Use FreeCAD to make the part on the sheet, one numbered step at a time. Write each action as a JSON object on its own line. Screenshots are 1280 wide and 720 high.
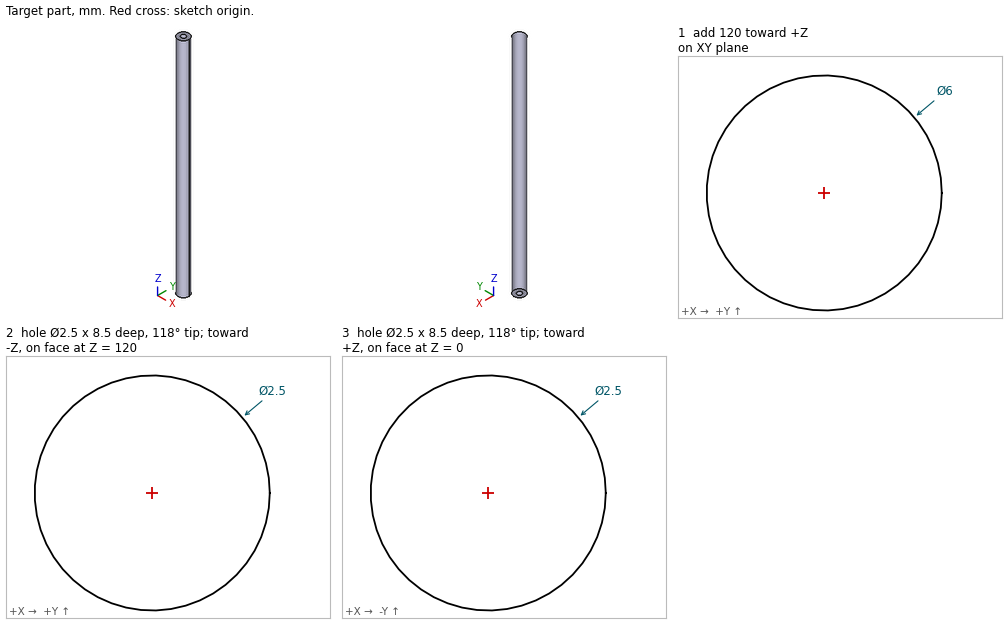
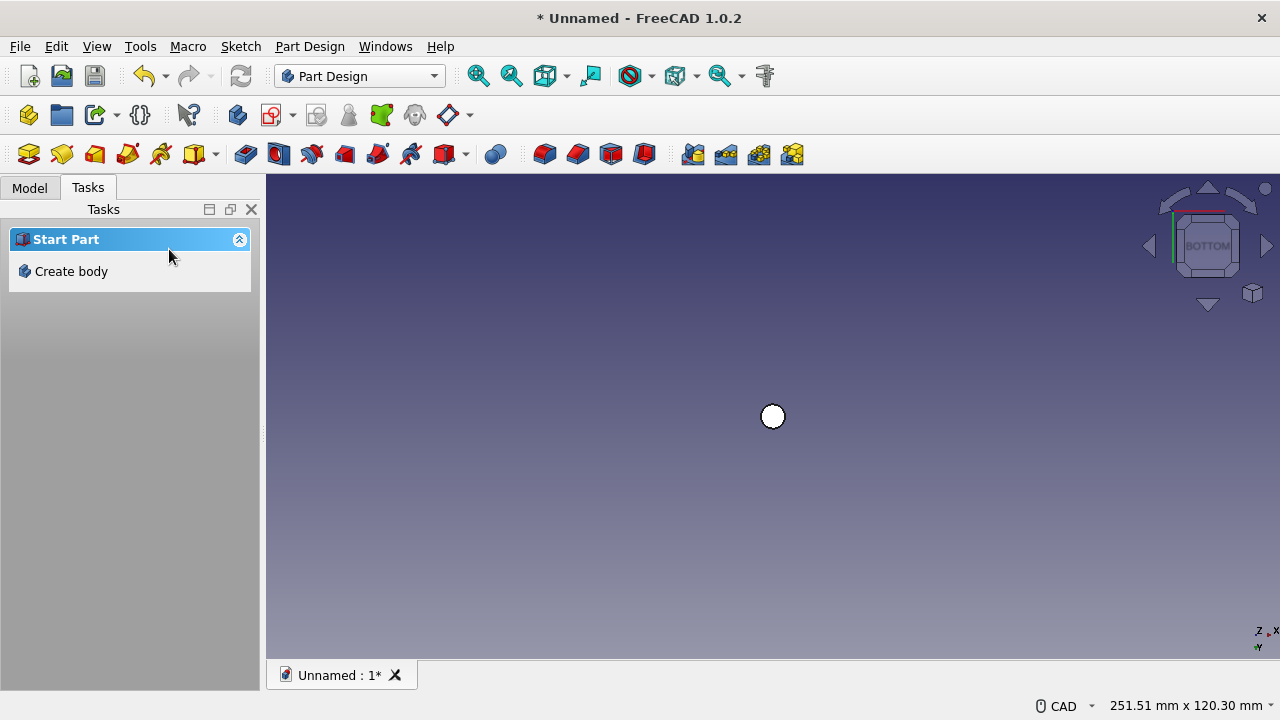
{"action": "left_click", "coordinate": [773, 415]}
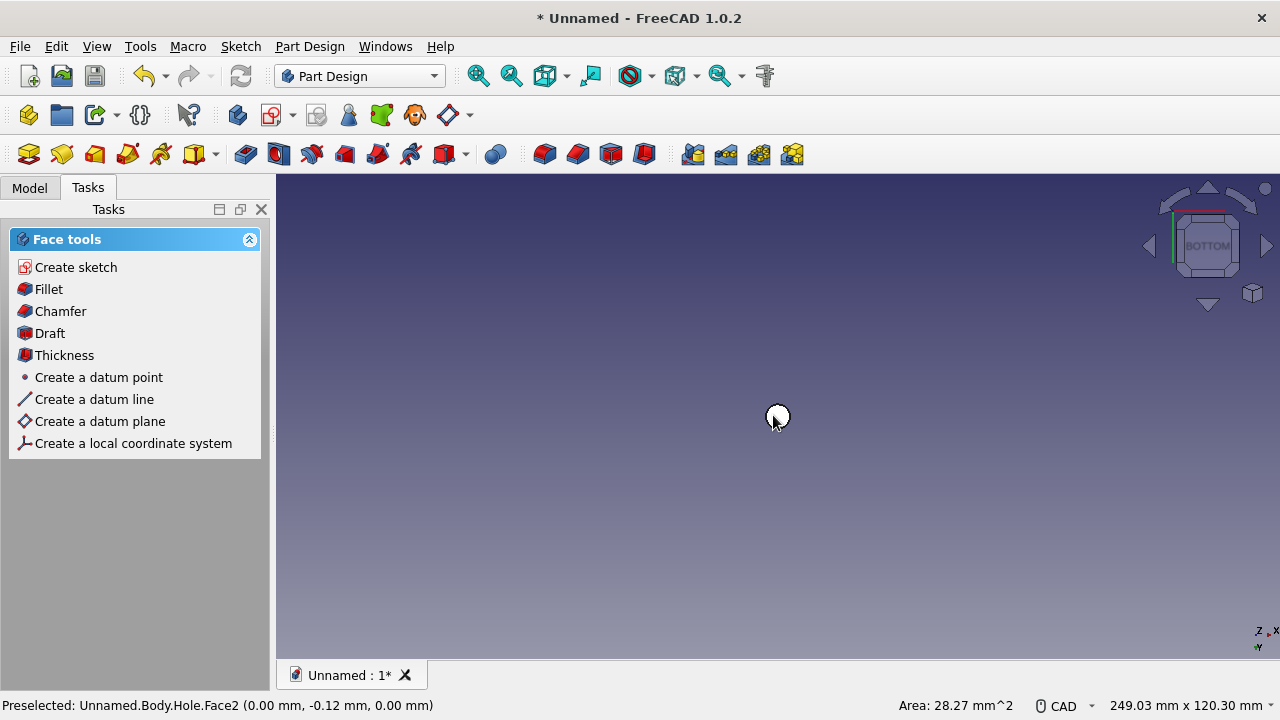
{"action": "left_click", "coordinate": [270, 116]}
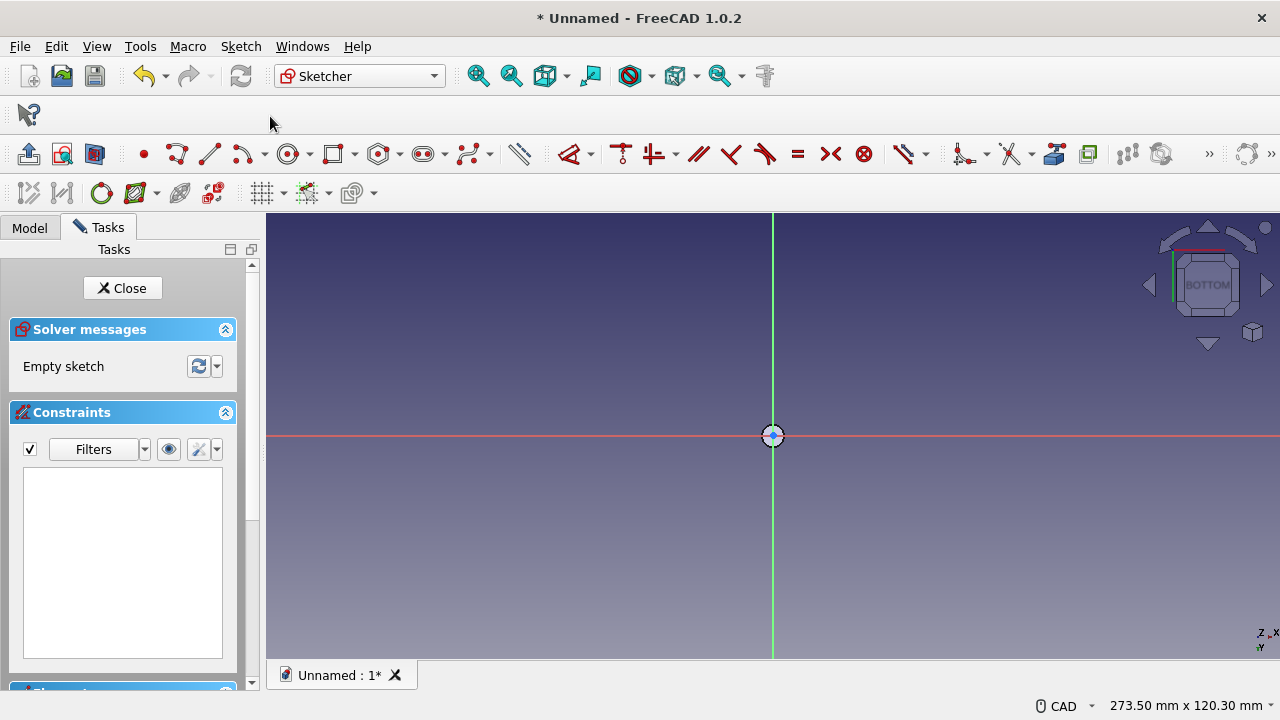
{"action": "scroll", "coordinate": [777, 436], "scroll_direction": "up", "scroll_amount": 15}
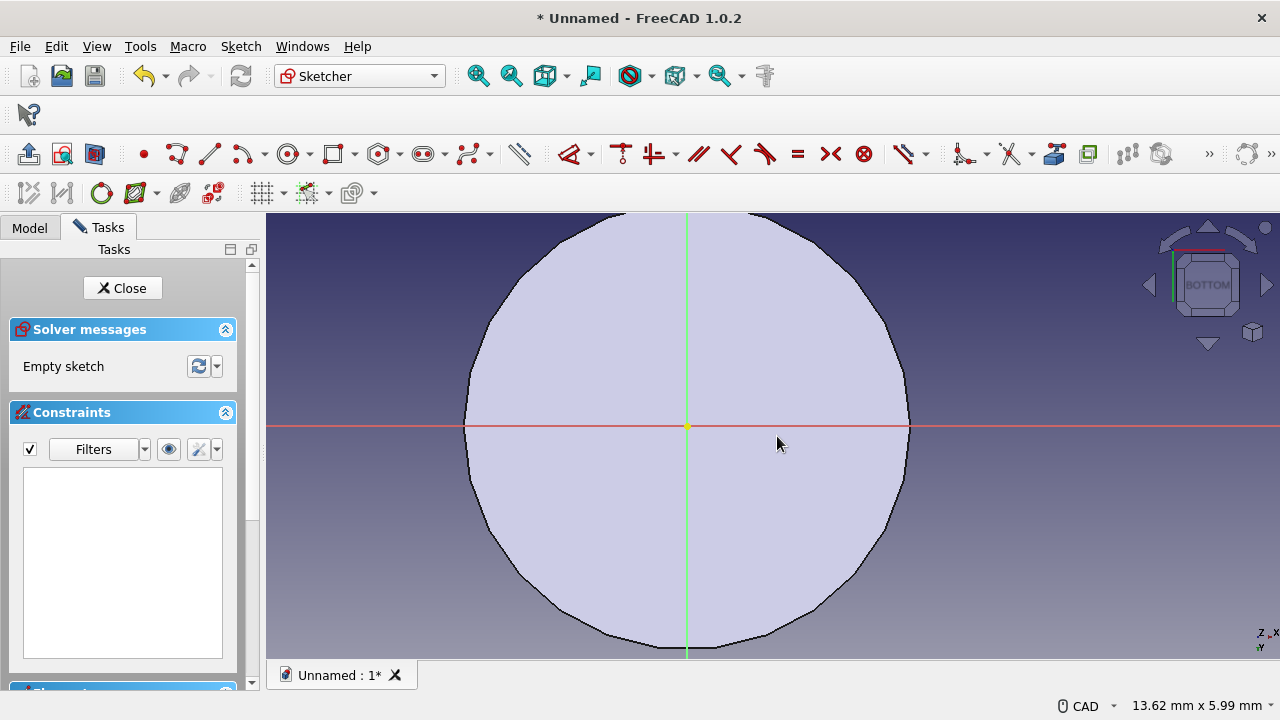
{"action": "scroll", "coordinate": [652, 407], "scroll_direction": "up", "scroll_amount": 2}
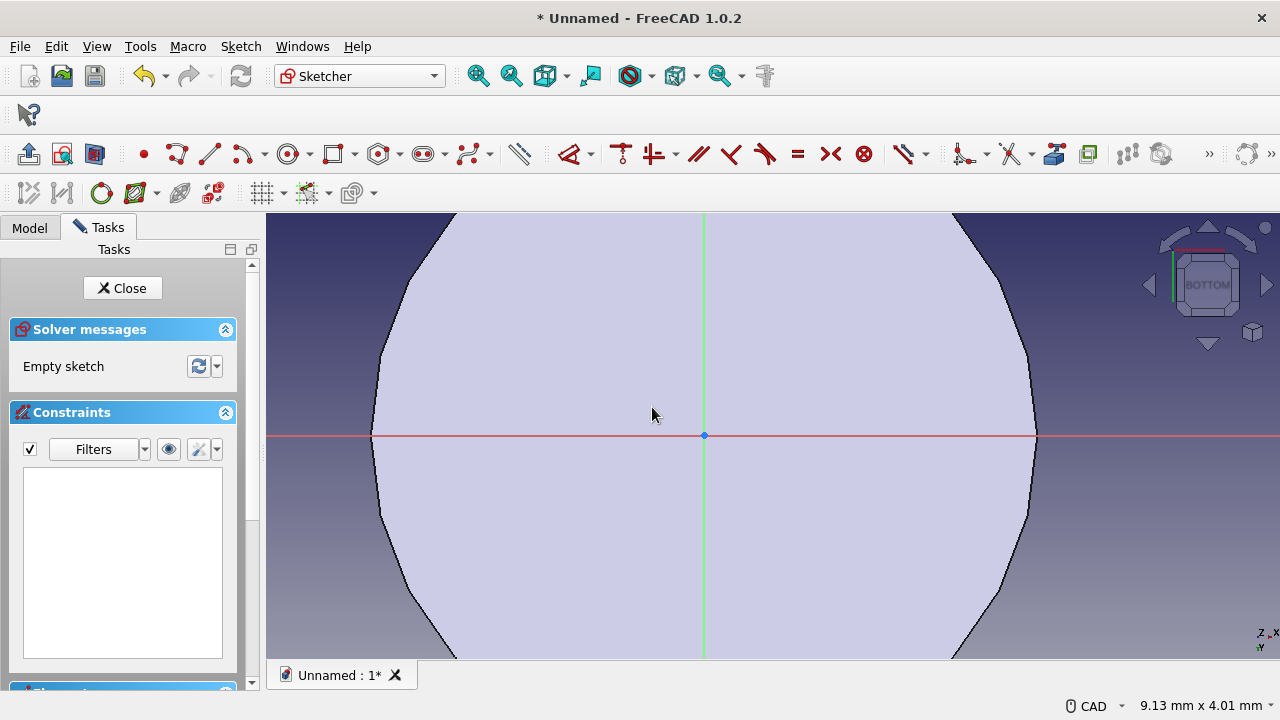
{"action": "key", "text": "g c"}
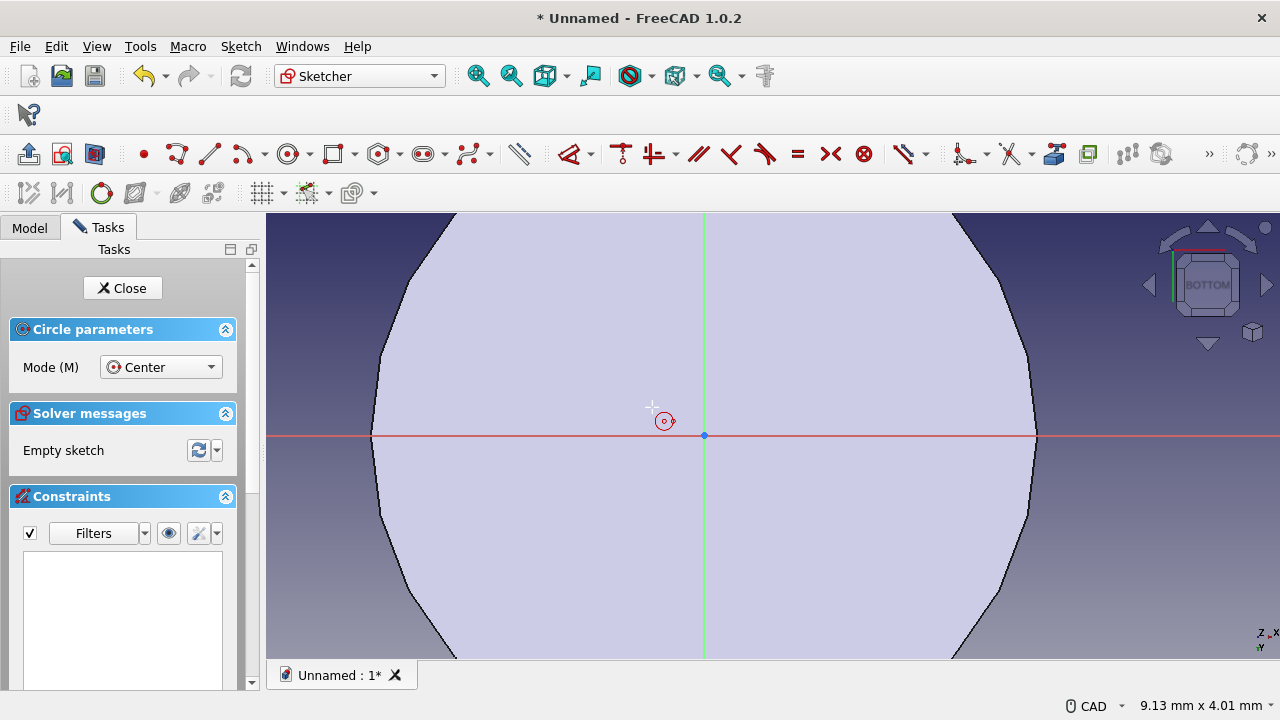
{"action": "left_click", "coordinate": [704, 436]}
{"action": "left_click", "coordinate": [802, 338]}
{"action": "key", "text": "Escape"}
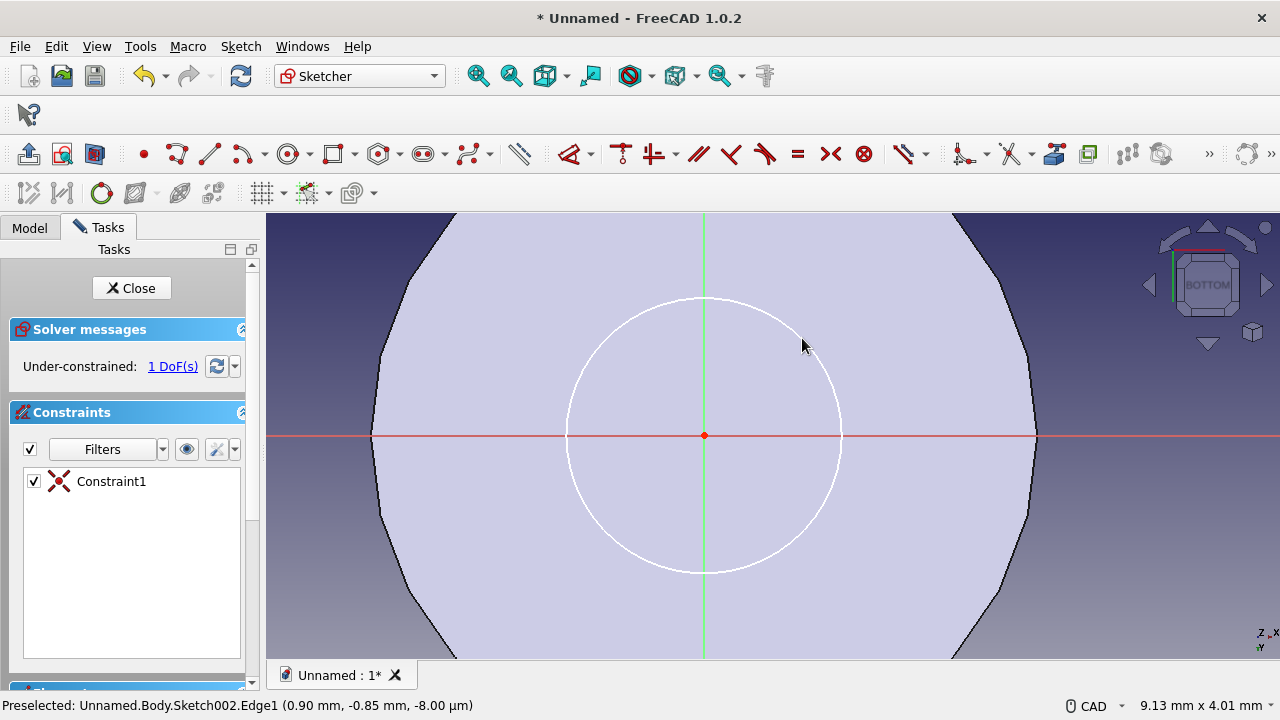
{"action": "key", "text": "d"}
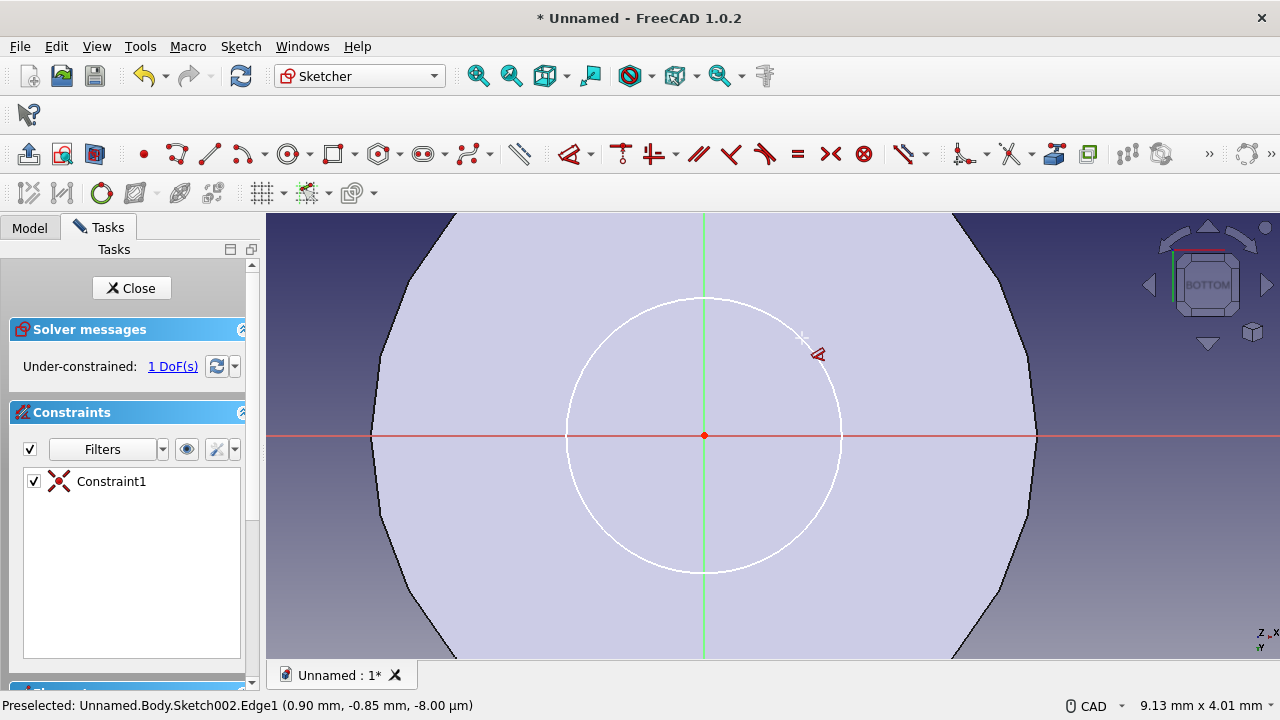
{"action": "left_click", "coordinate": [801, 338]}
{"action": "left_click", "coordinate": [824, 315]}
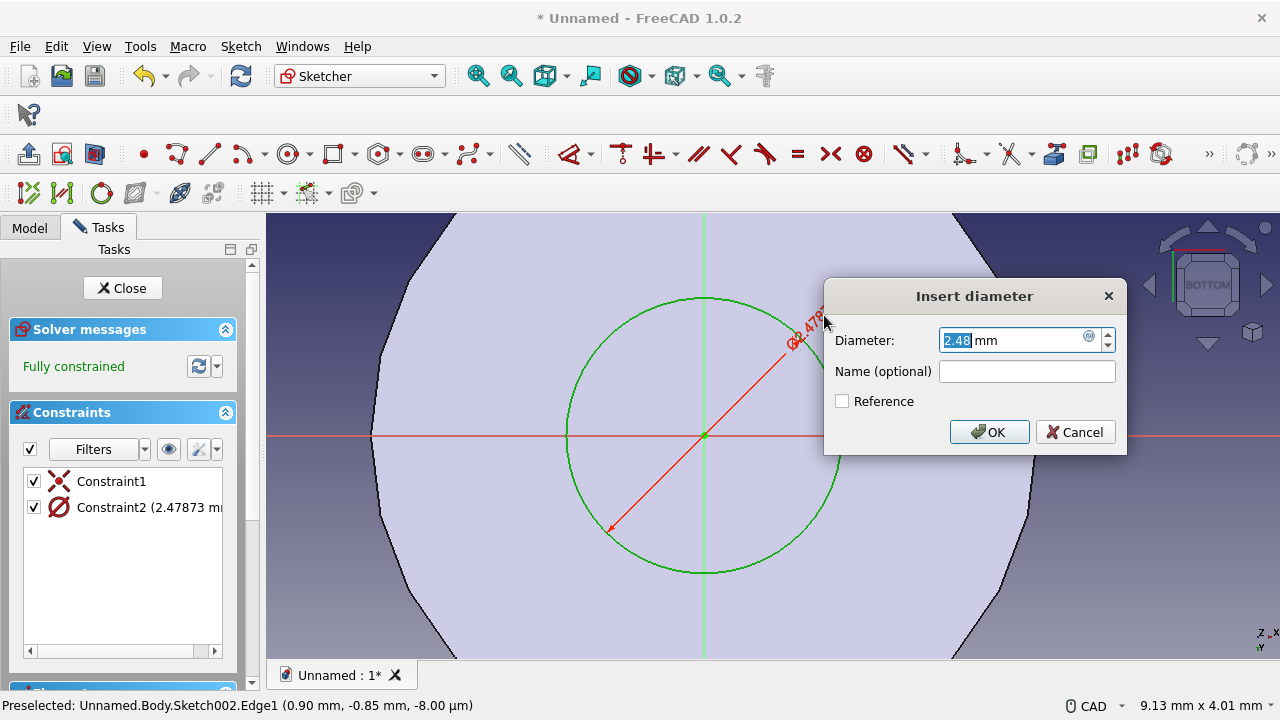
{"action": "type", "text": "2.5"}
{"action": "key", "text": "Return"}
{"action": "key", "text": "Escape"}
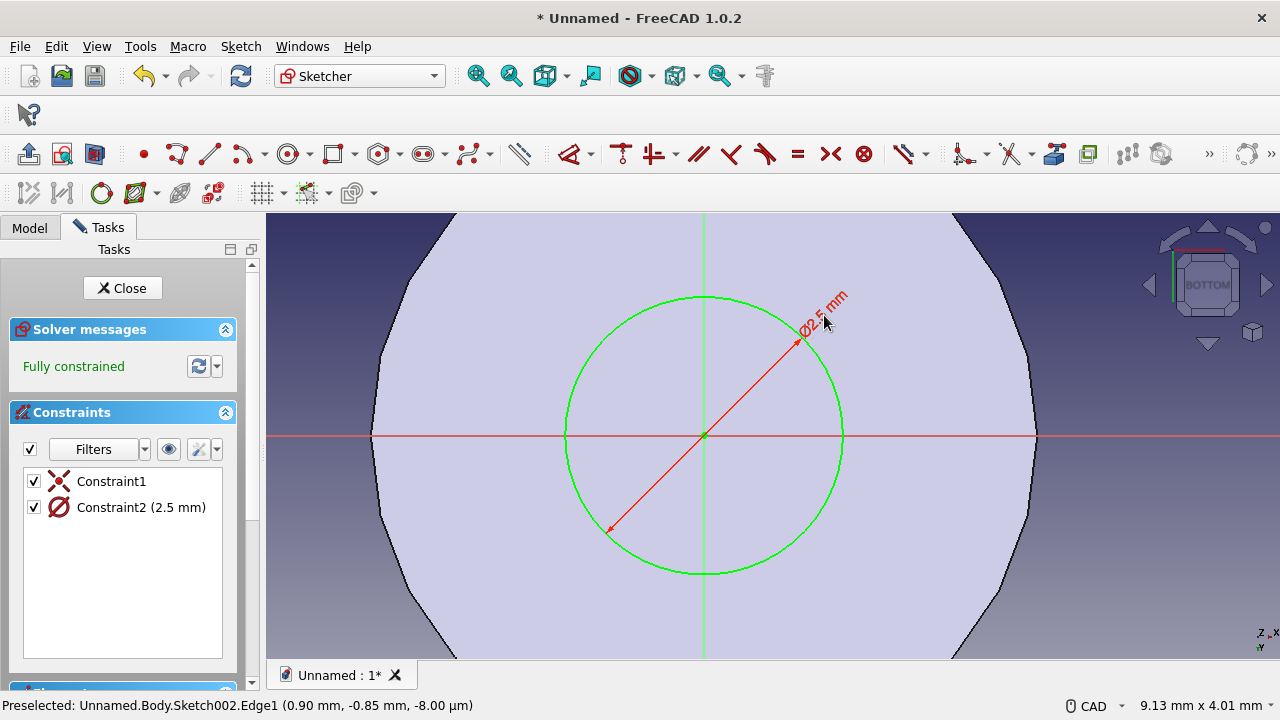
{"action": "left_click", "coordinate": [123, 288]}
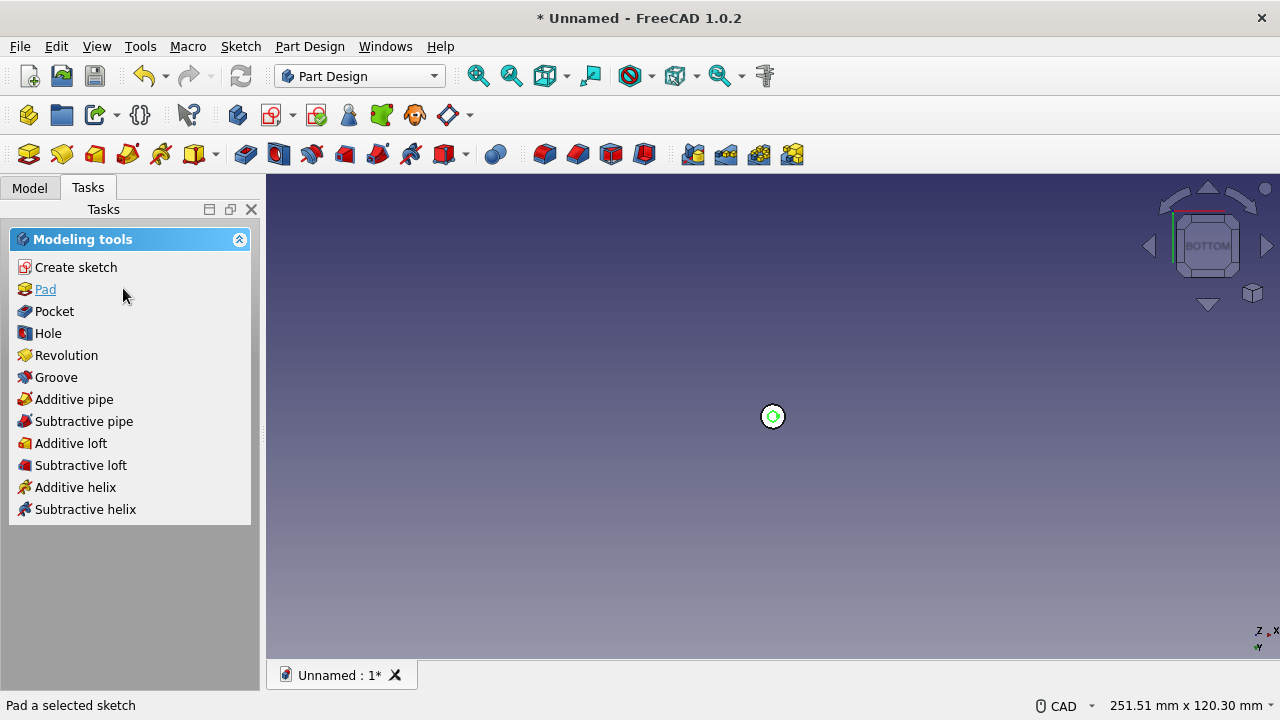
{"action": "left_click", "coordinate": [279, 154]}